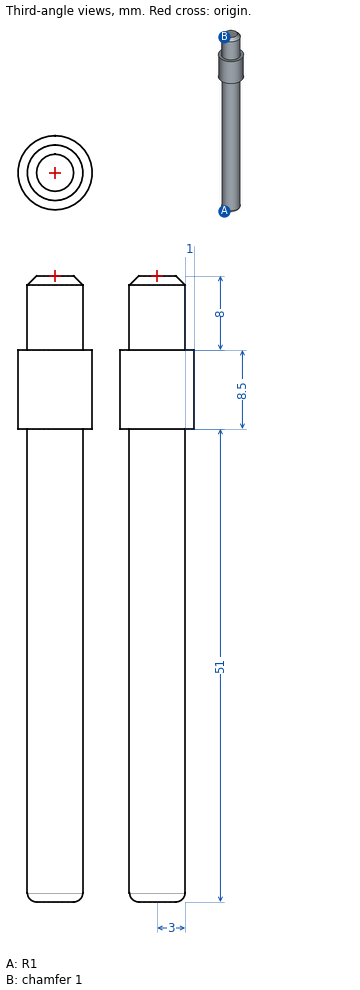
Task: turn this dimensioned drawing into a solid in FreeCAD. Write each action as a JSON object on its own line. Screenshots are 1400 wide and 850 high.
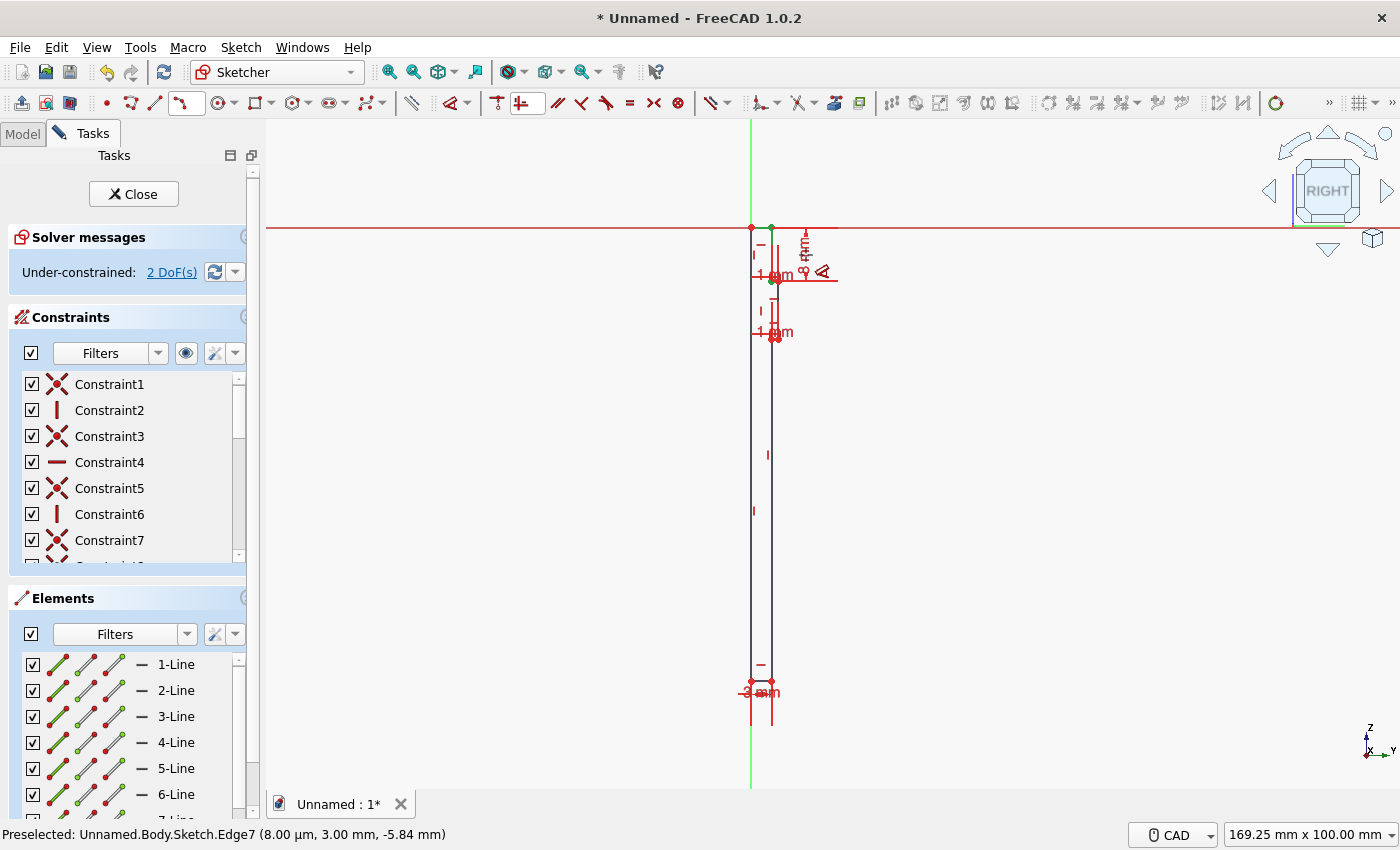
{"action": "left_click", "coordinate": [772, 579]}
{"action": "left_click", "coordinate": [806, 510]}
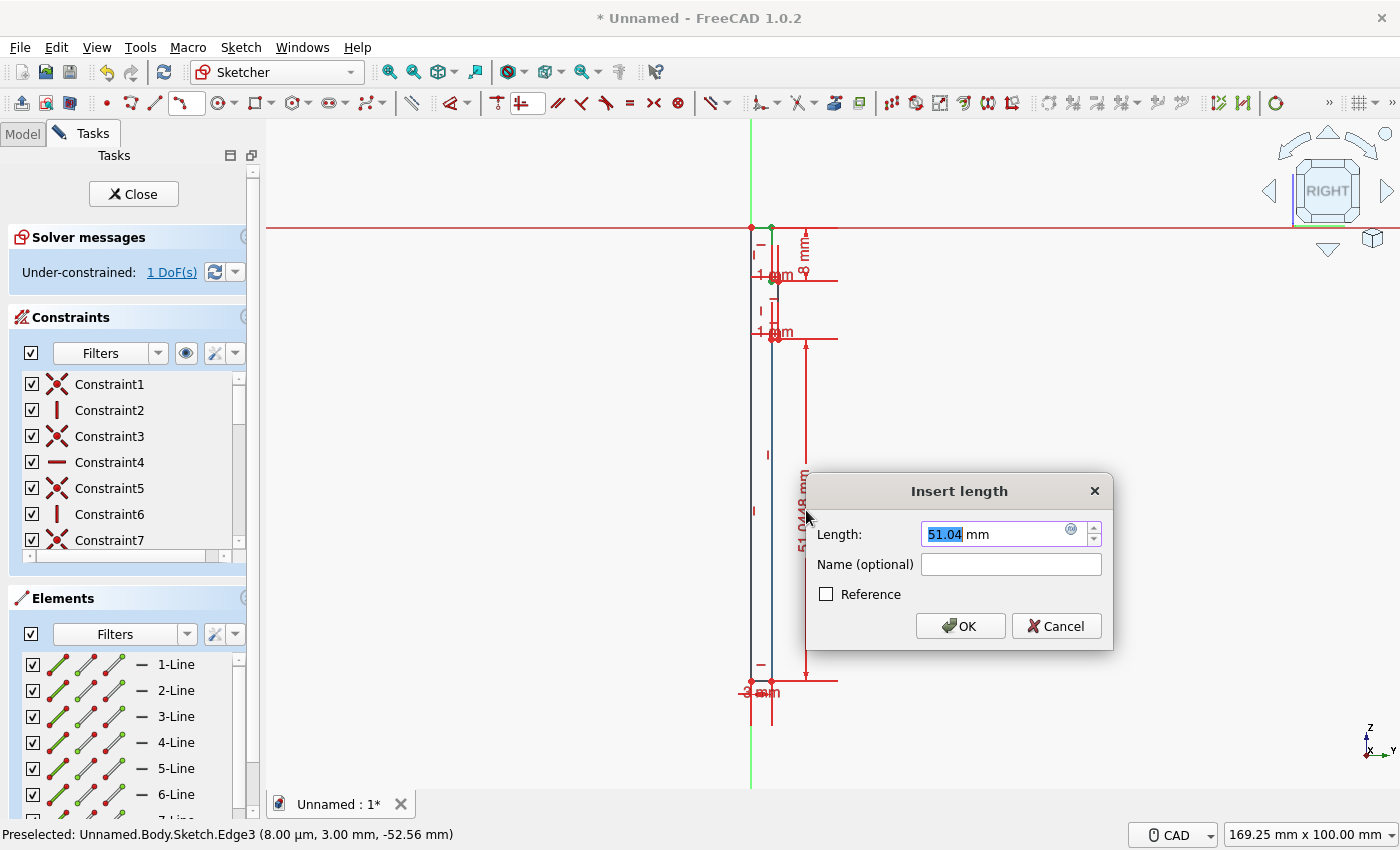
{"action": "type", "text": "51"}
{"action": "key", "text": "Return"}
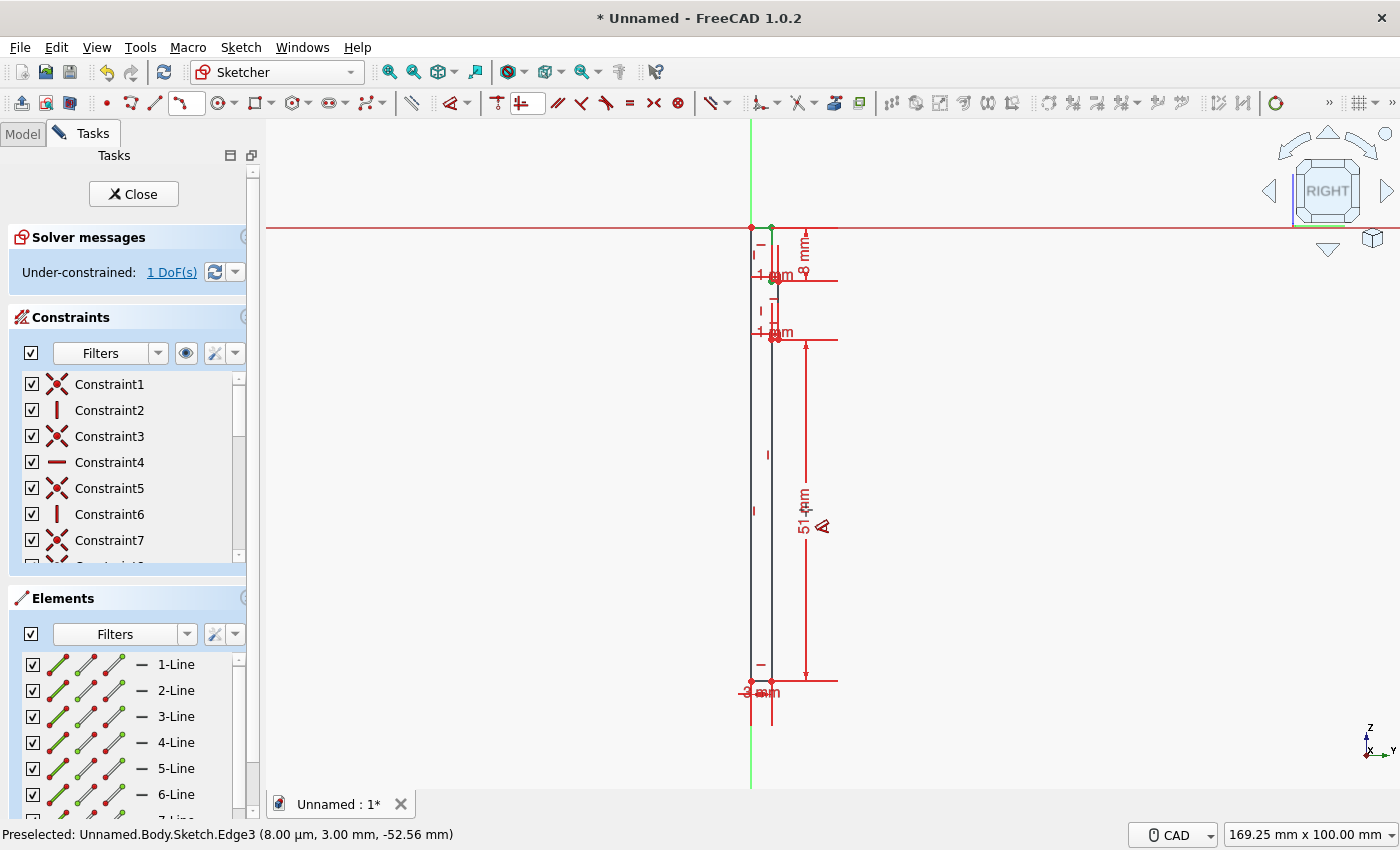
{"action": "left_click", "coordinate": [778, 322]}
{"action": "left_click", "coordinate": [812, 311]}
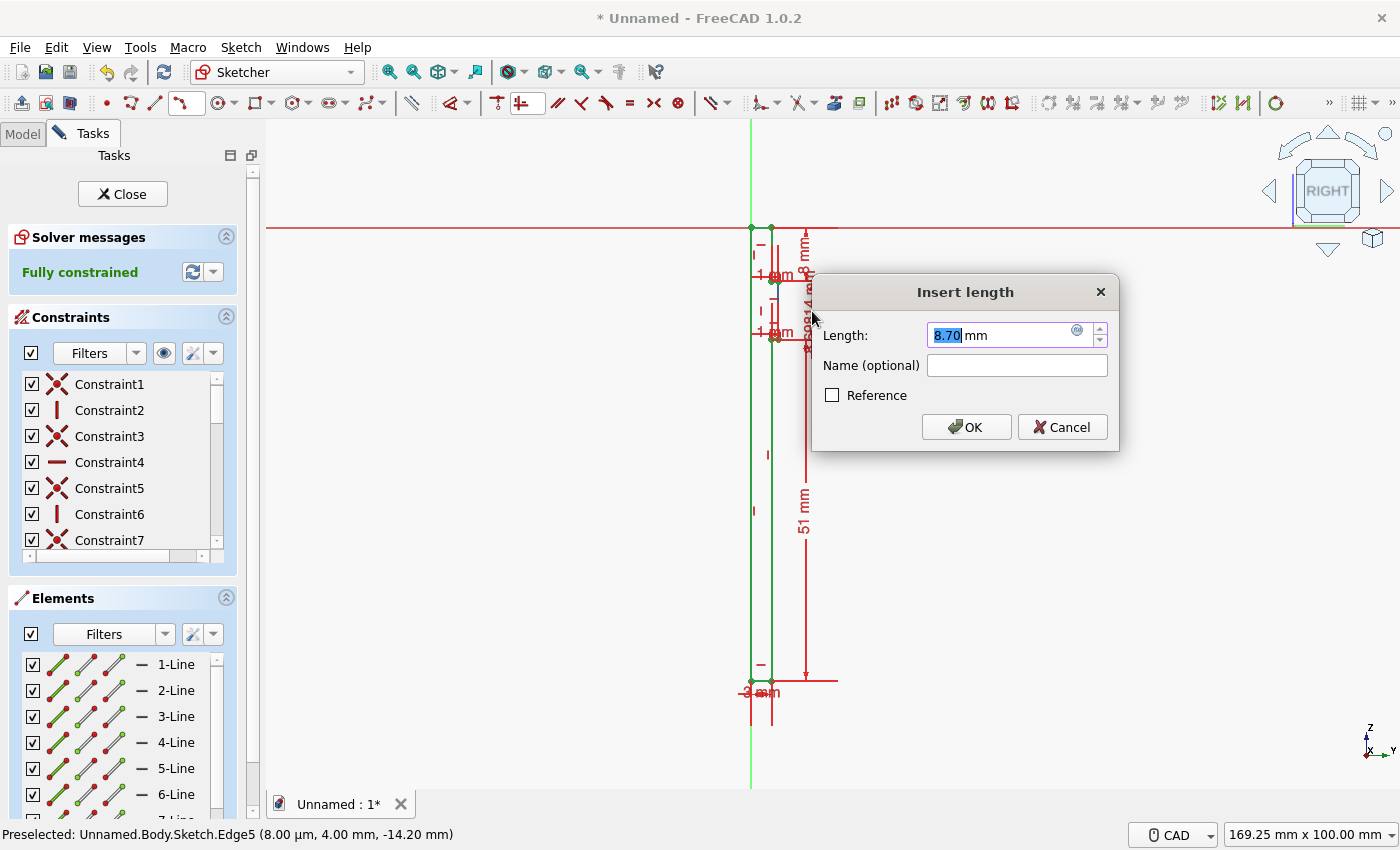
{"action": "type", "text": "8.5"}
{"action": "key", "text": "Return"}
{"action": "key", "text": "Escape"}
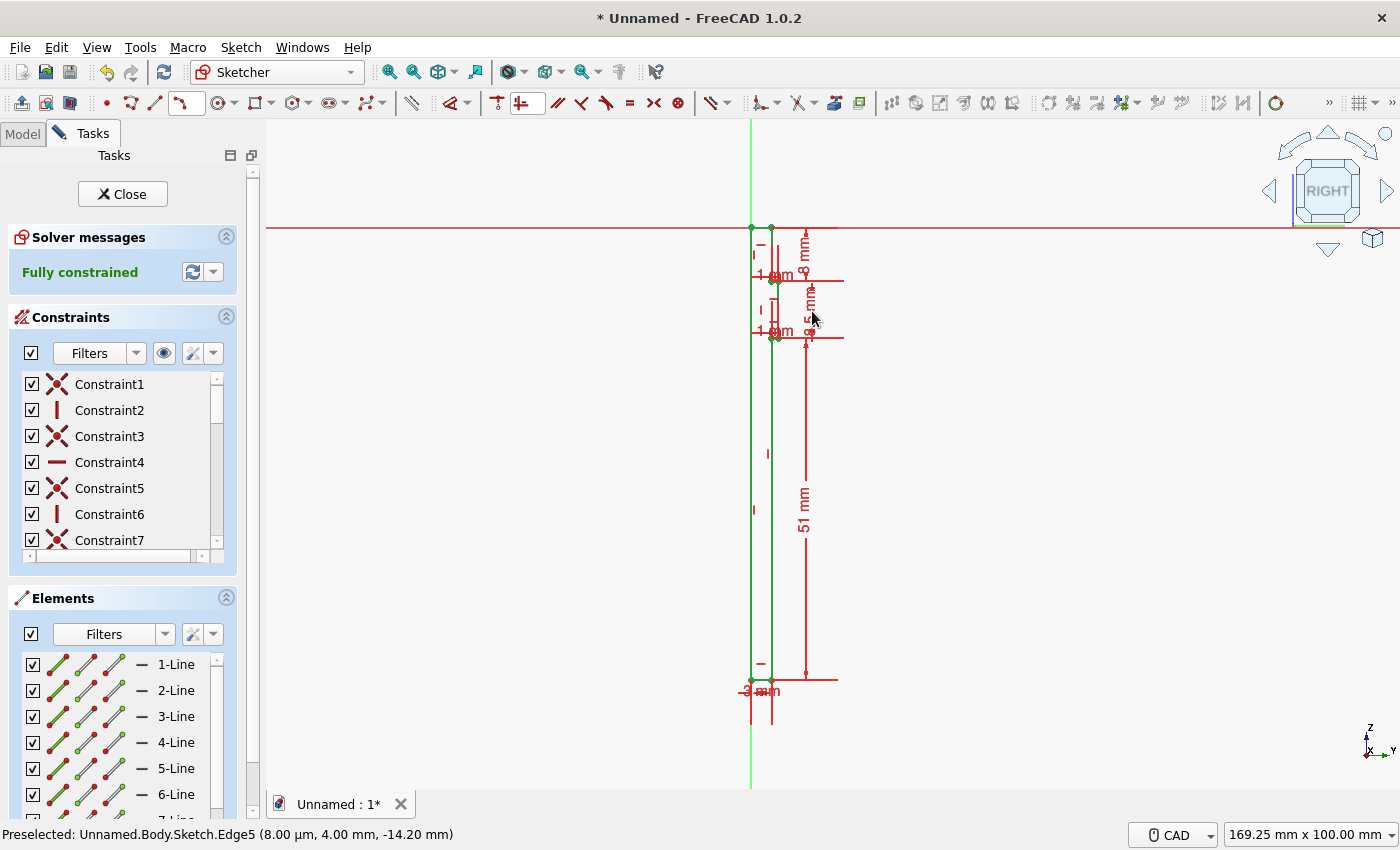
{"action": "left_click", "coordinate": [123, 194]}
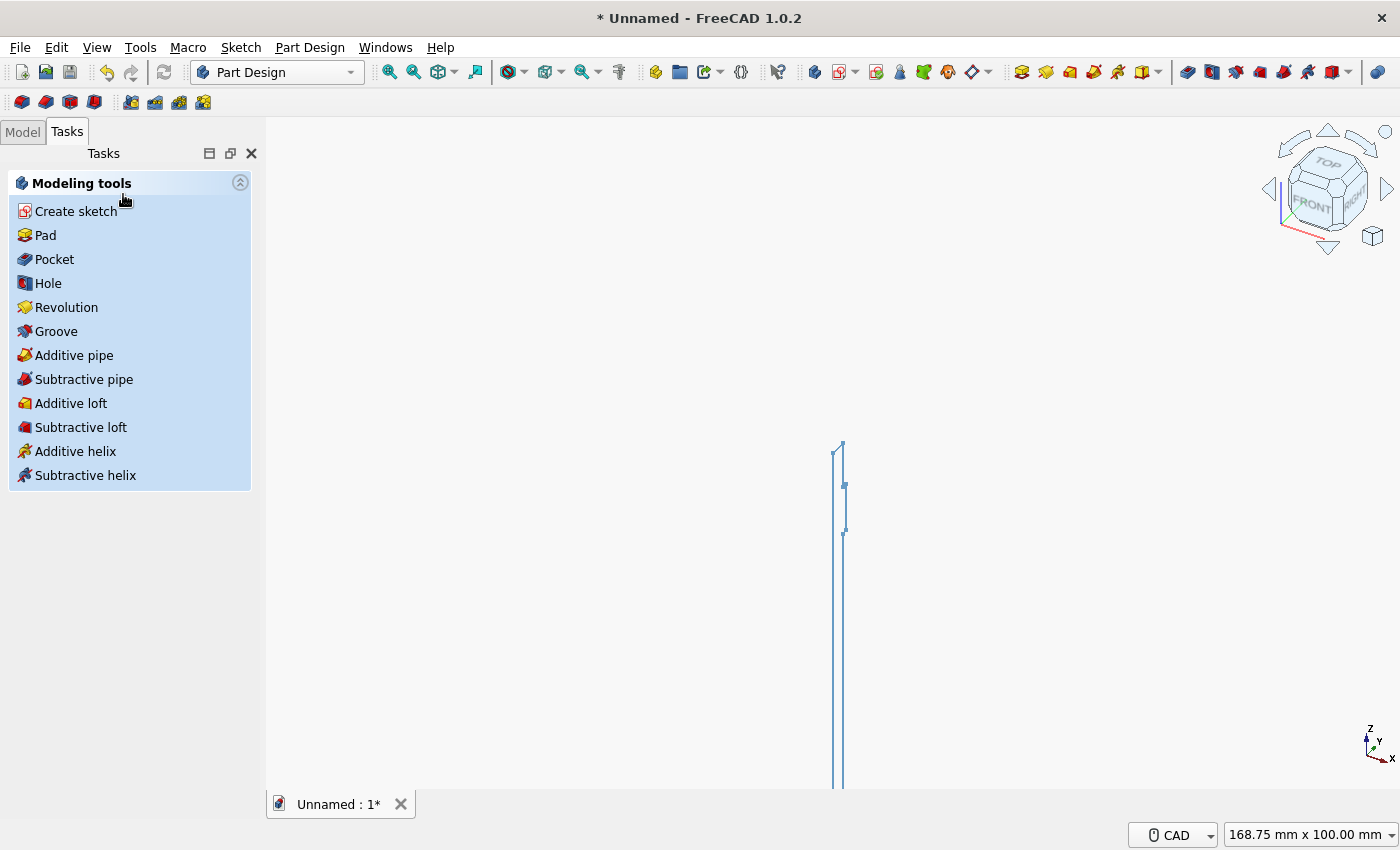
{"action": "left_click", "coordinate": [1046, 72]}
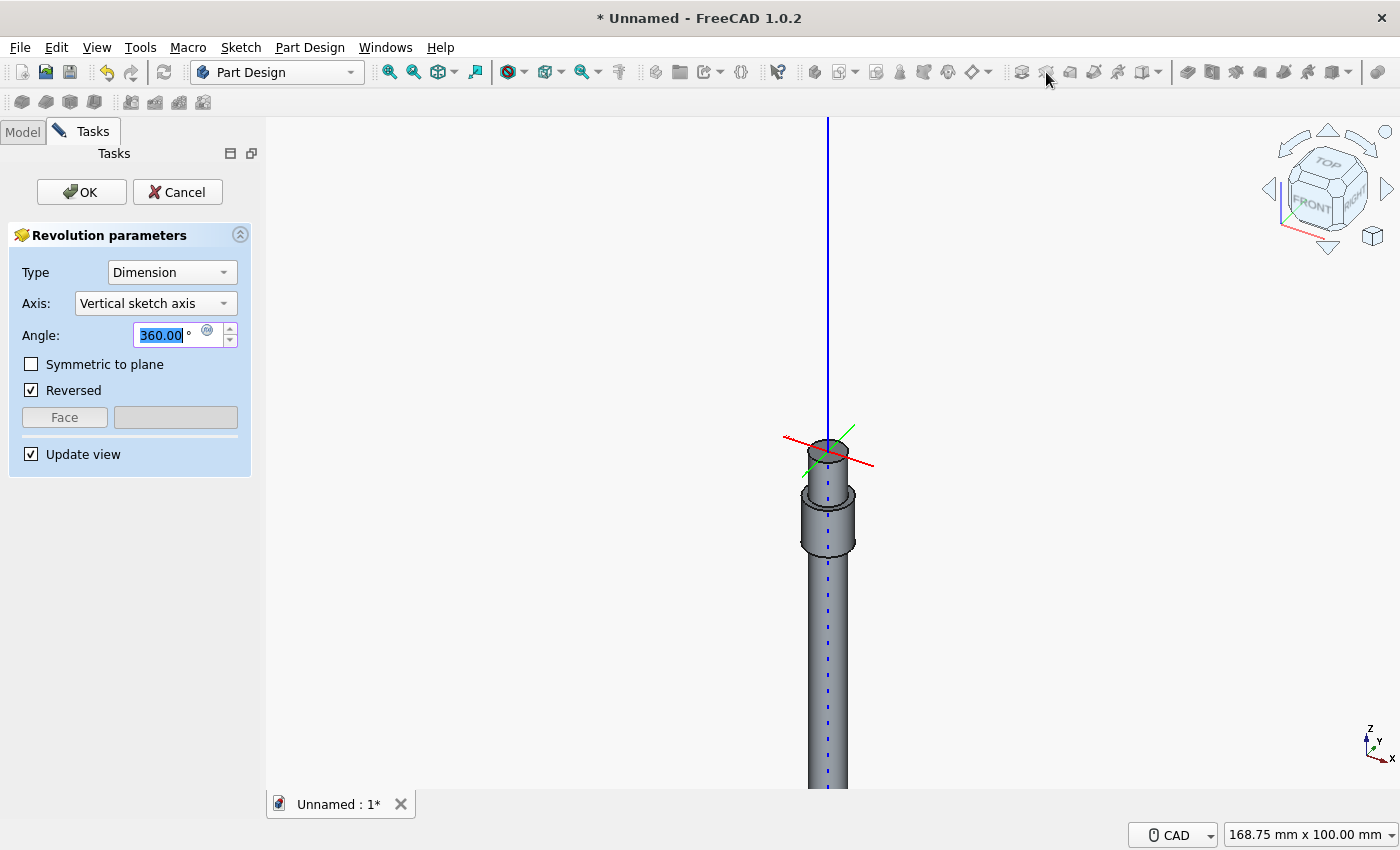
{"action": "left_click", "coordinate": [82, 192]}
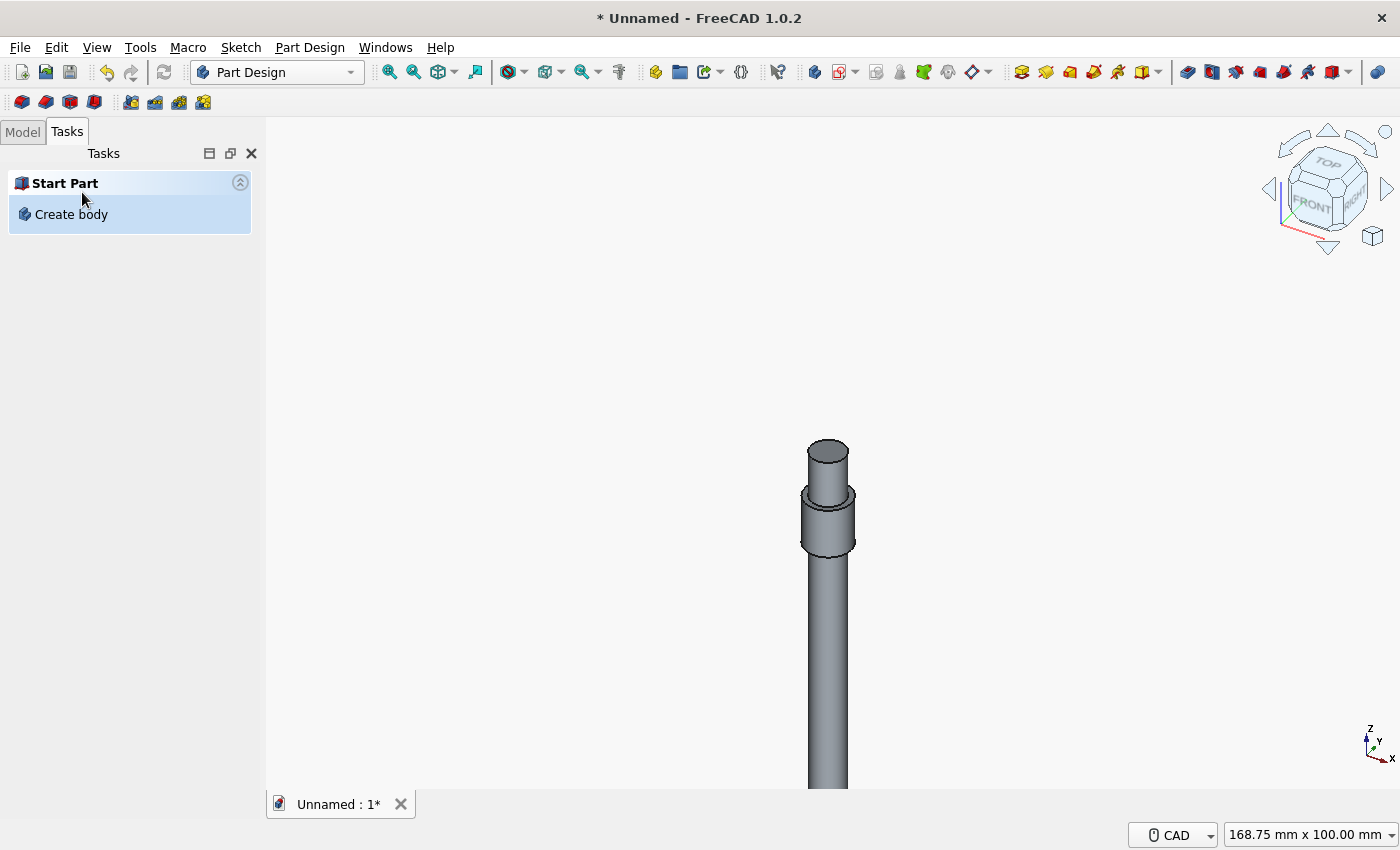
{"action": "left_click", "coordinate": [390, 72]}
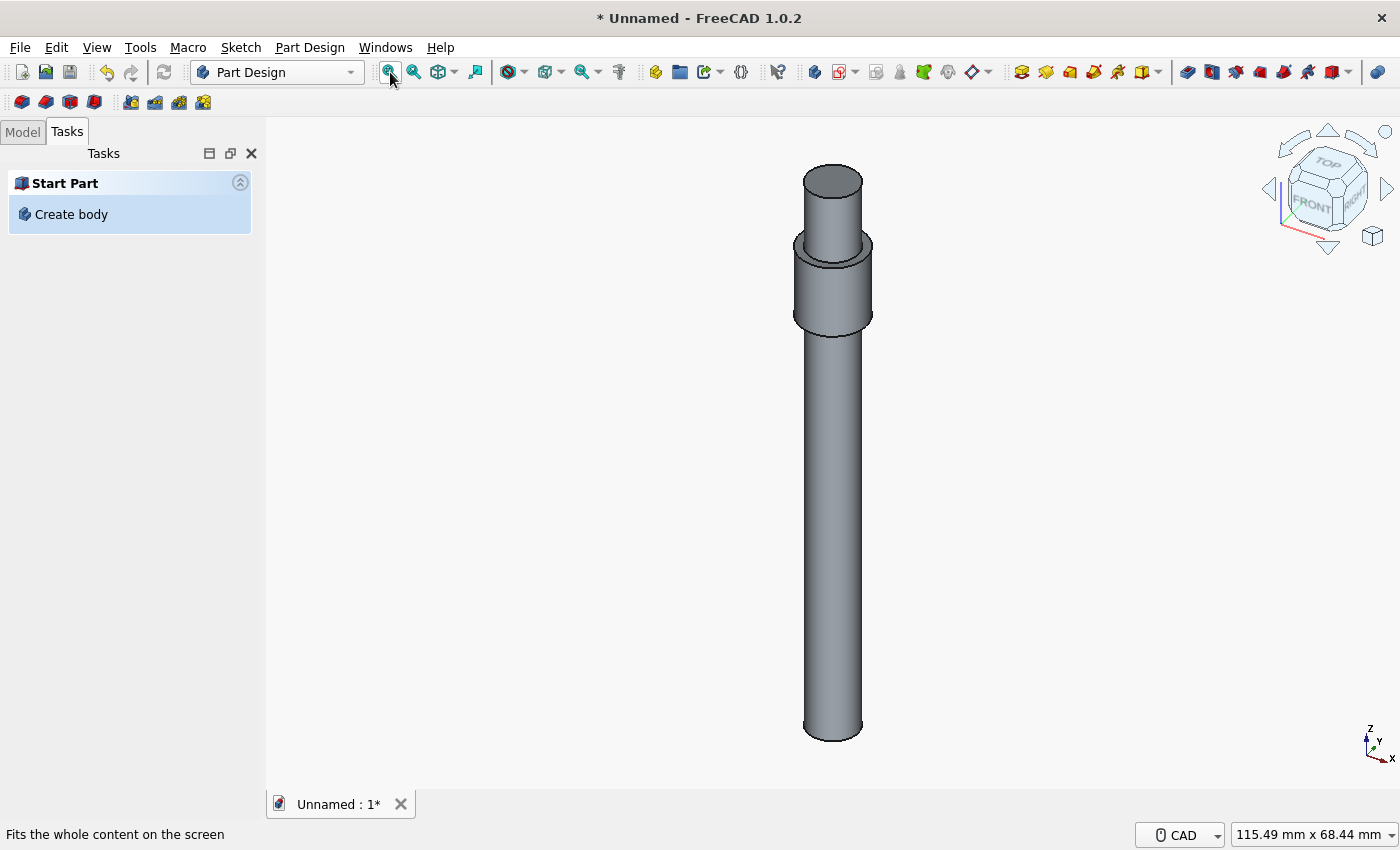
{"action": "left_click", "coordinate": [806, 730]}